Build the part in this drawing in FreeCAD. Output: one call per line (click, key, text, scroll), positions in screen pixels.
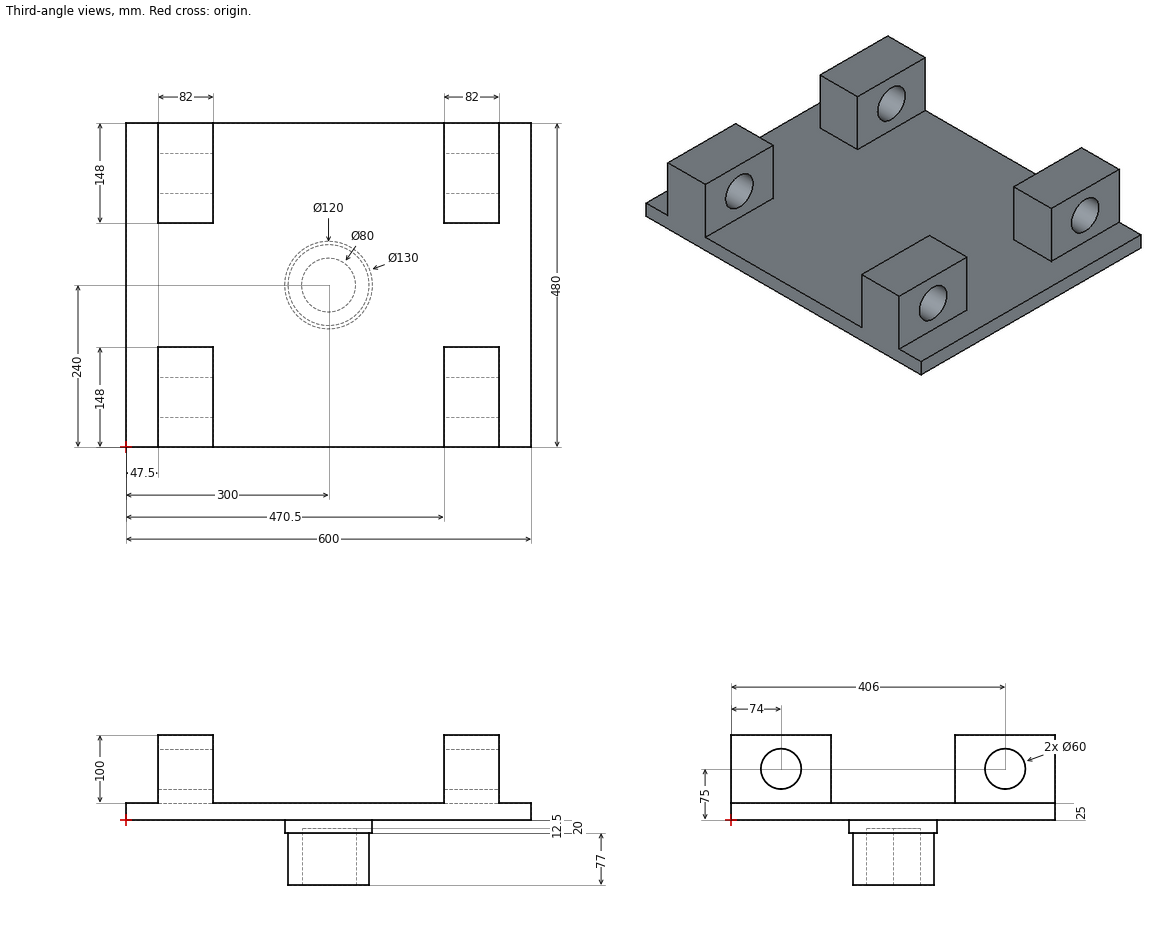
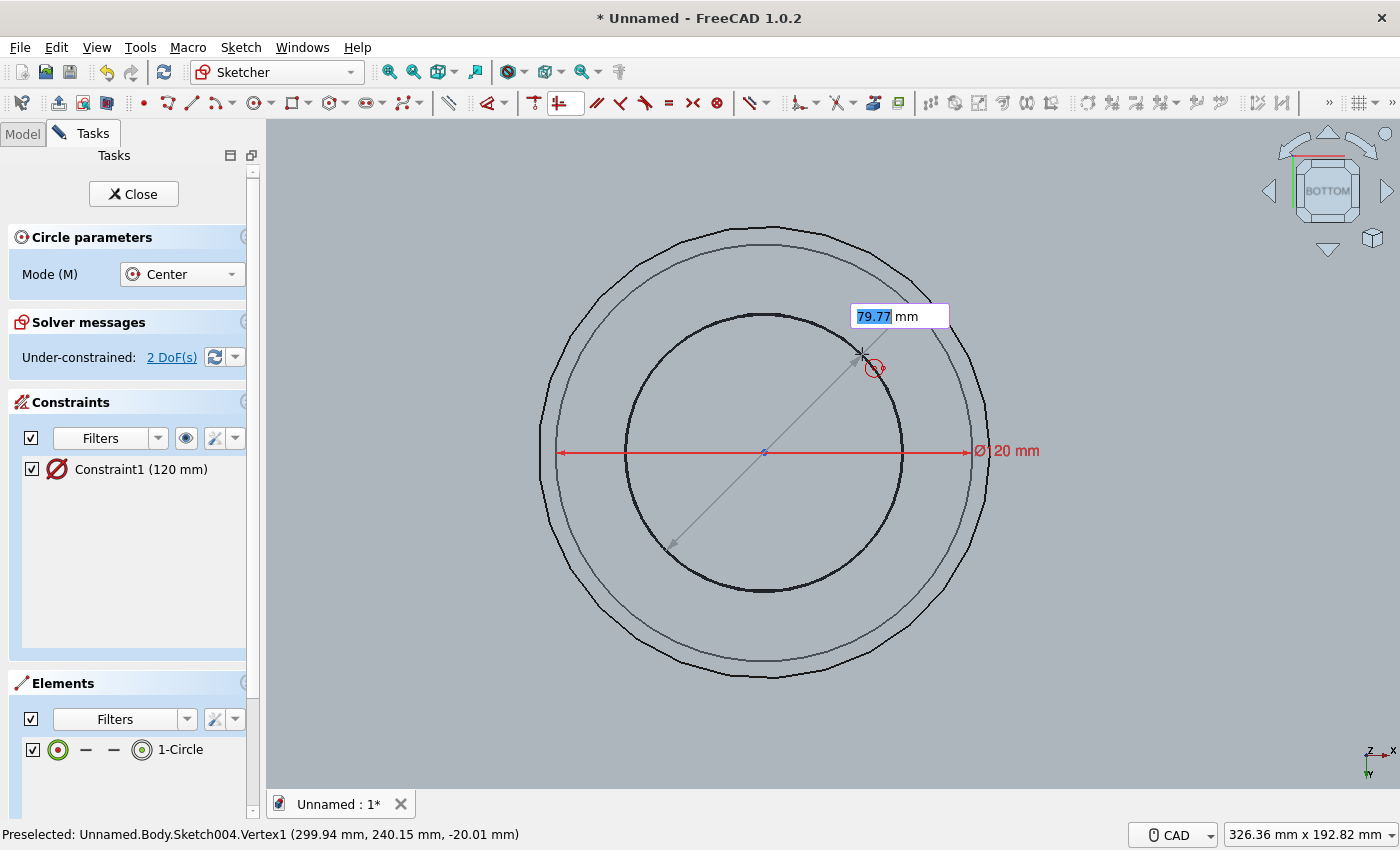
text(80)
key(Return)
key(Escape)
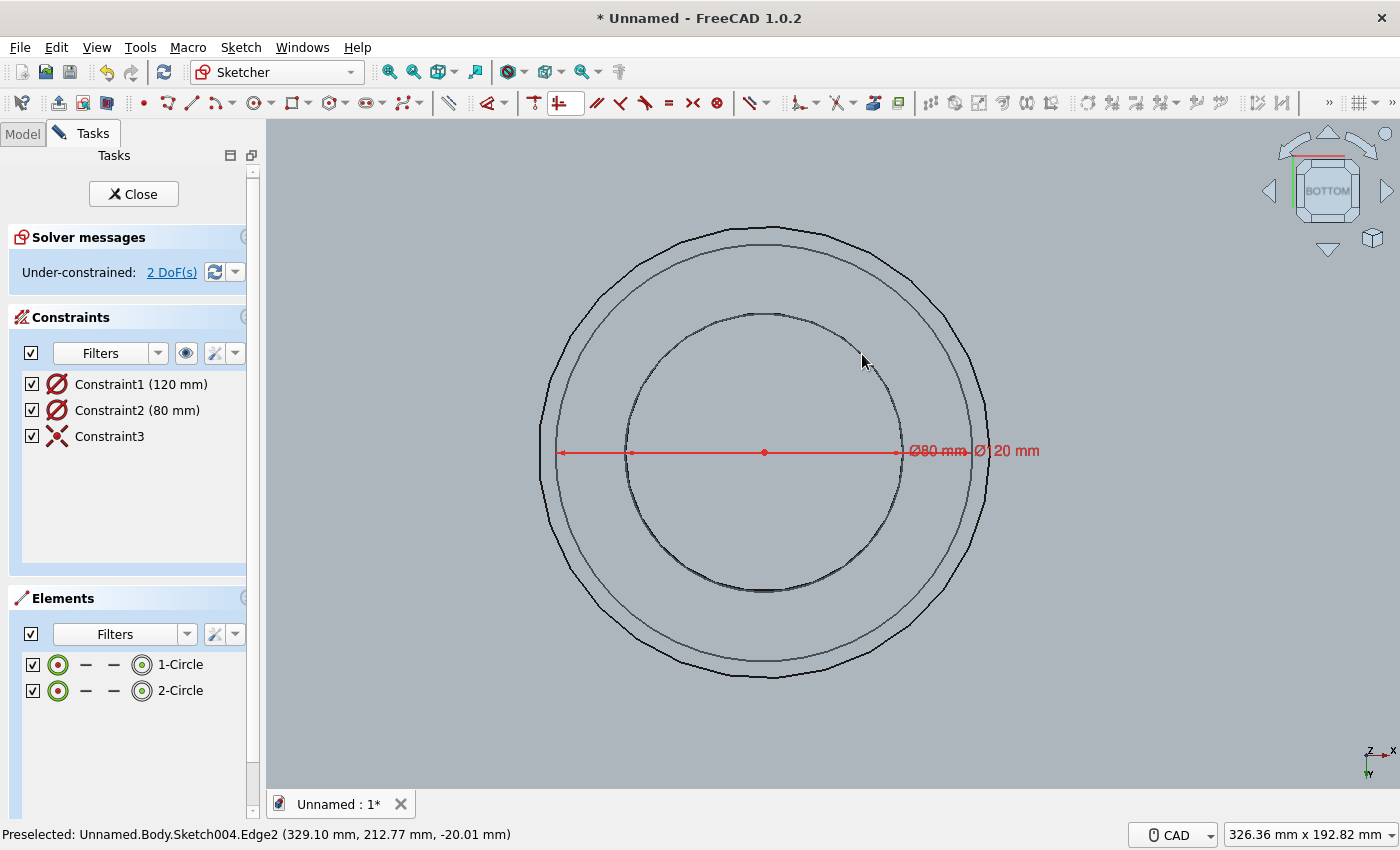
key(d)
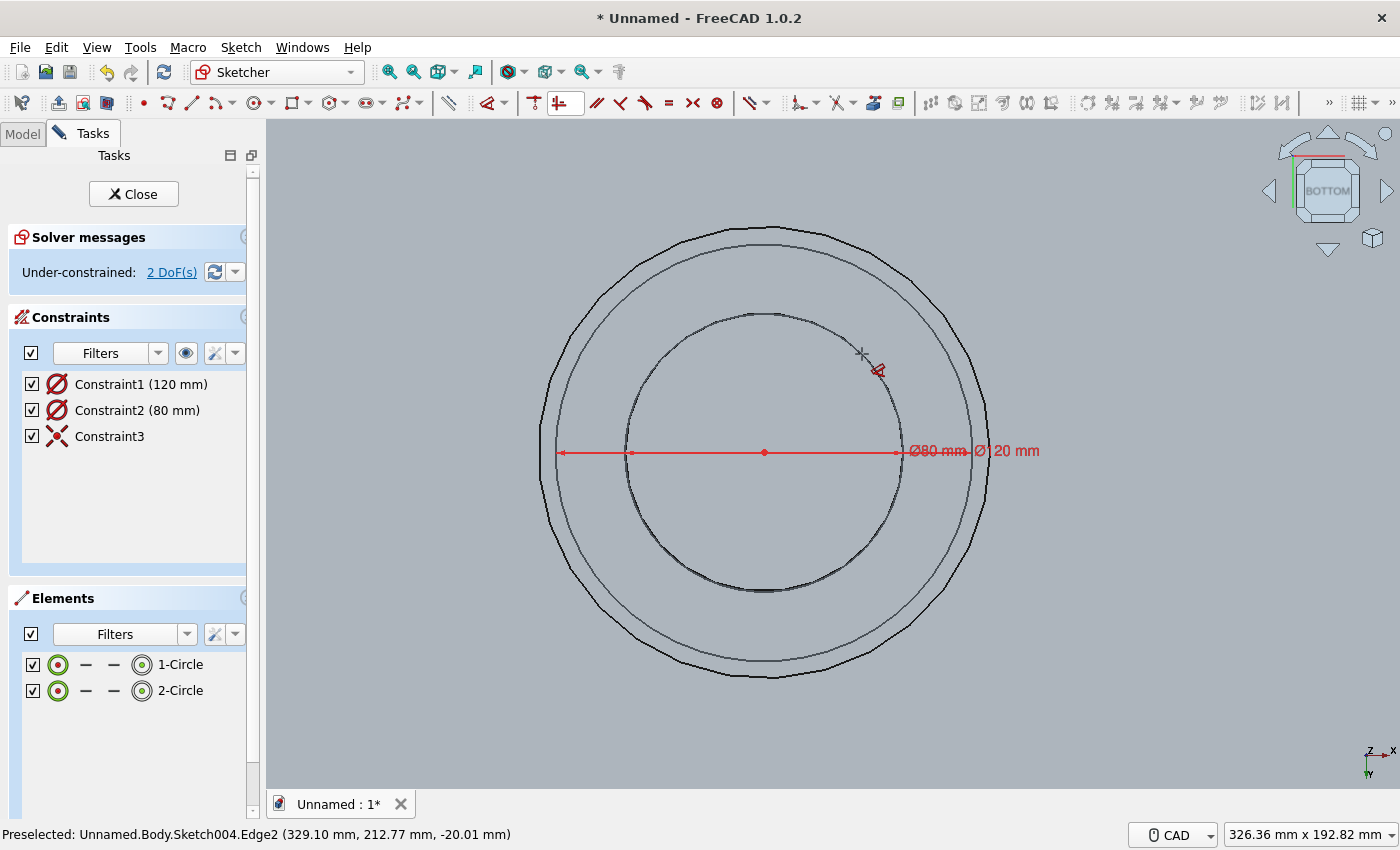
click(764, 453)
click(529, 487)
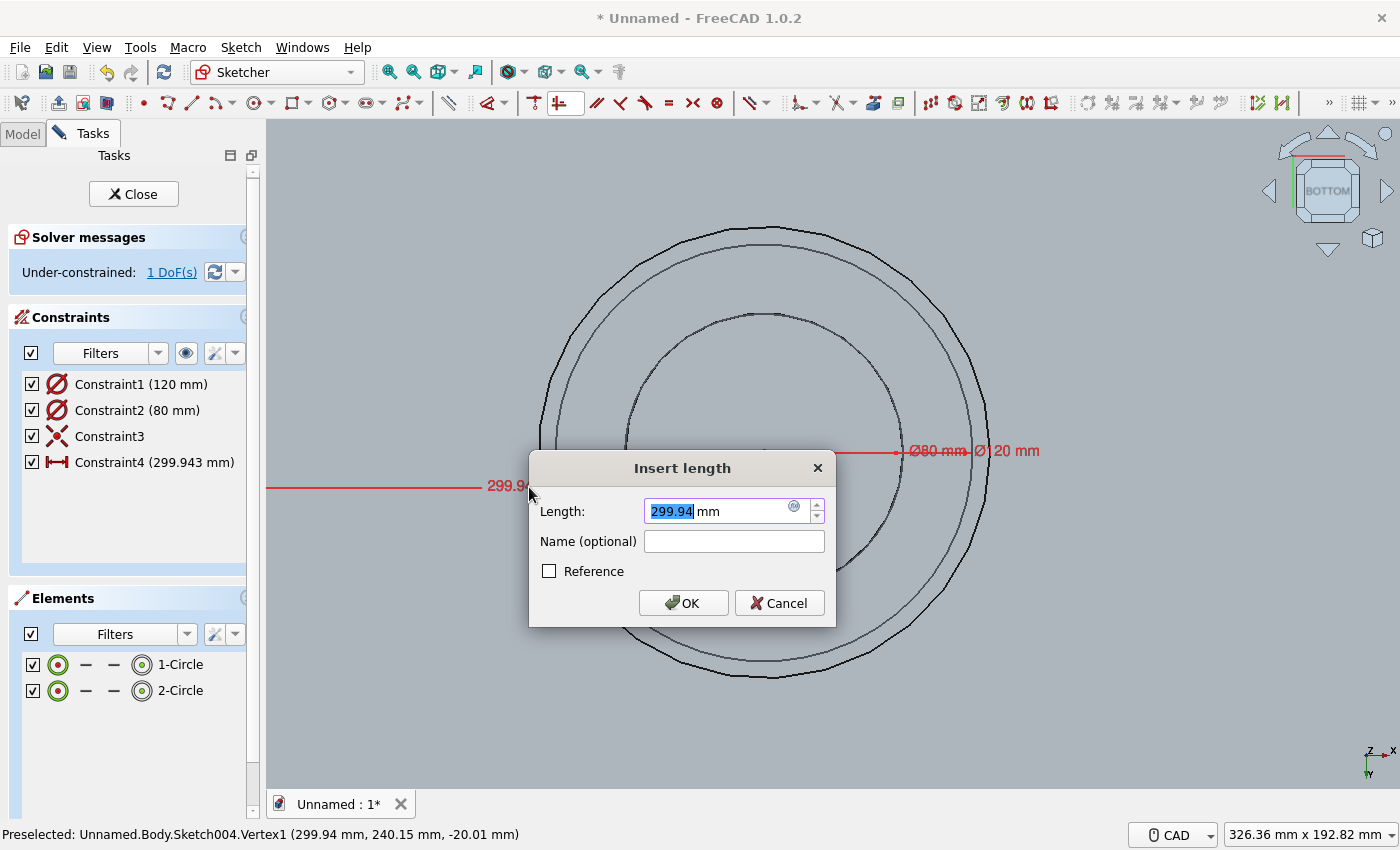
text(300)
key(Return)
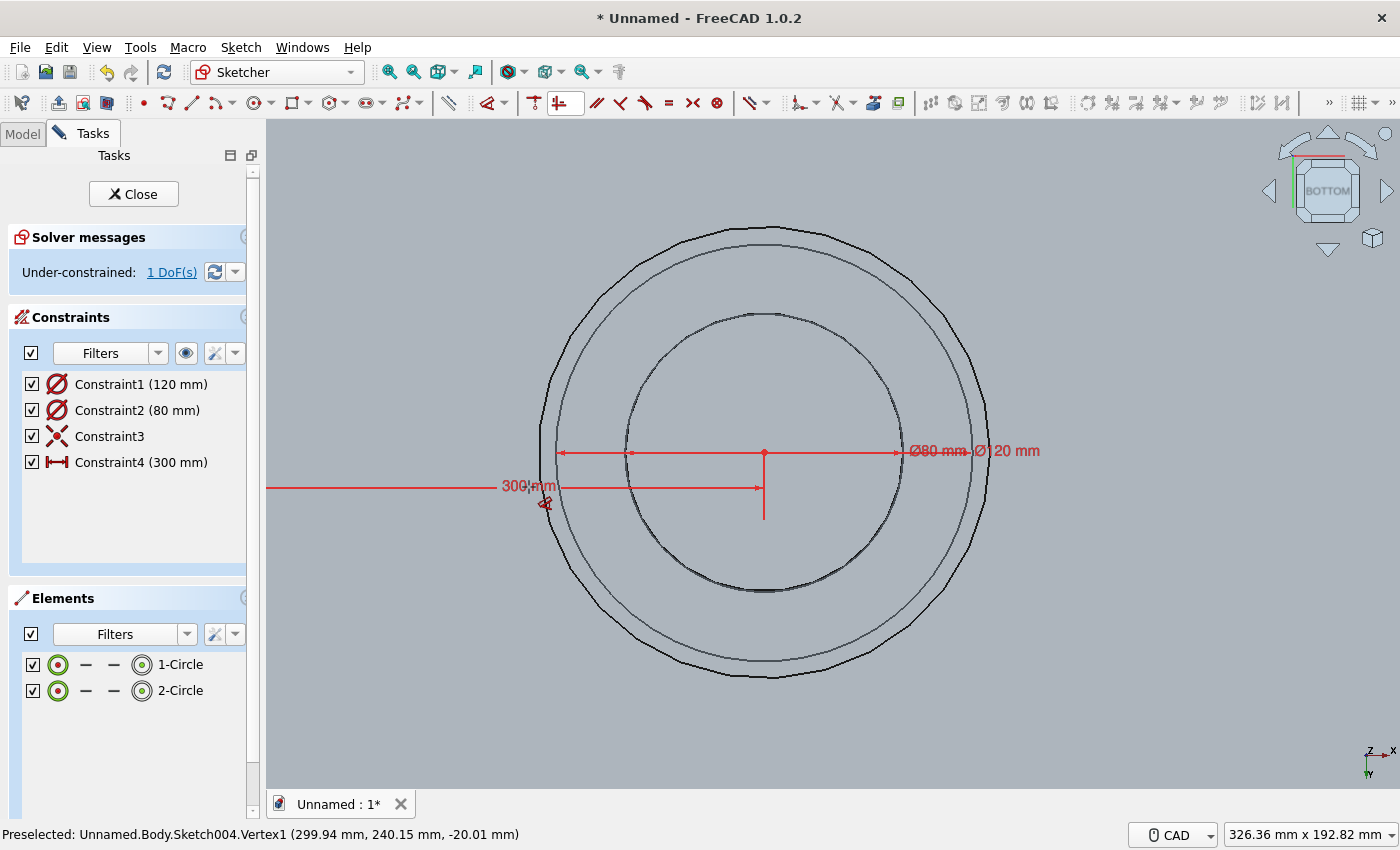
click(764, 453)
click(798, 300)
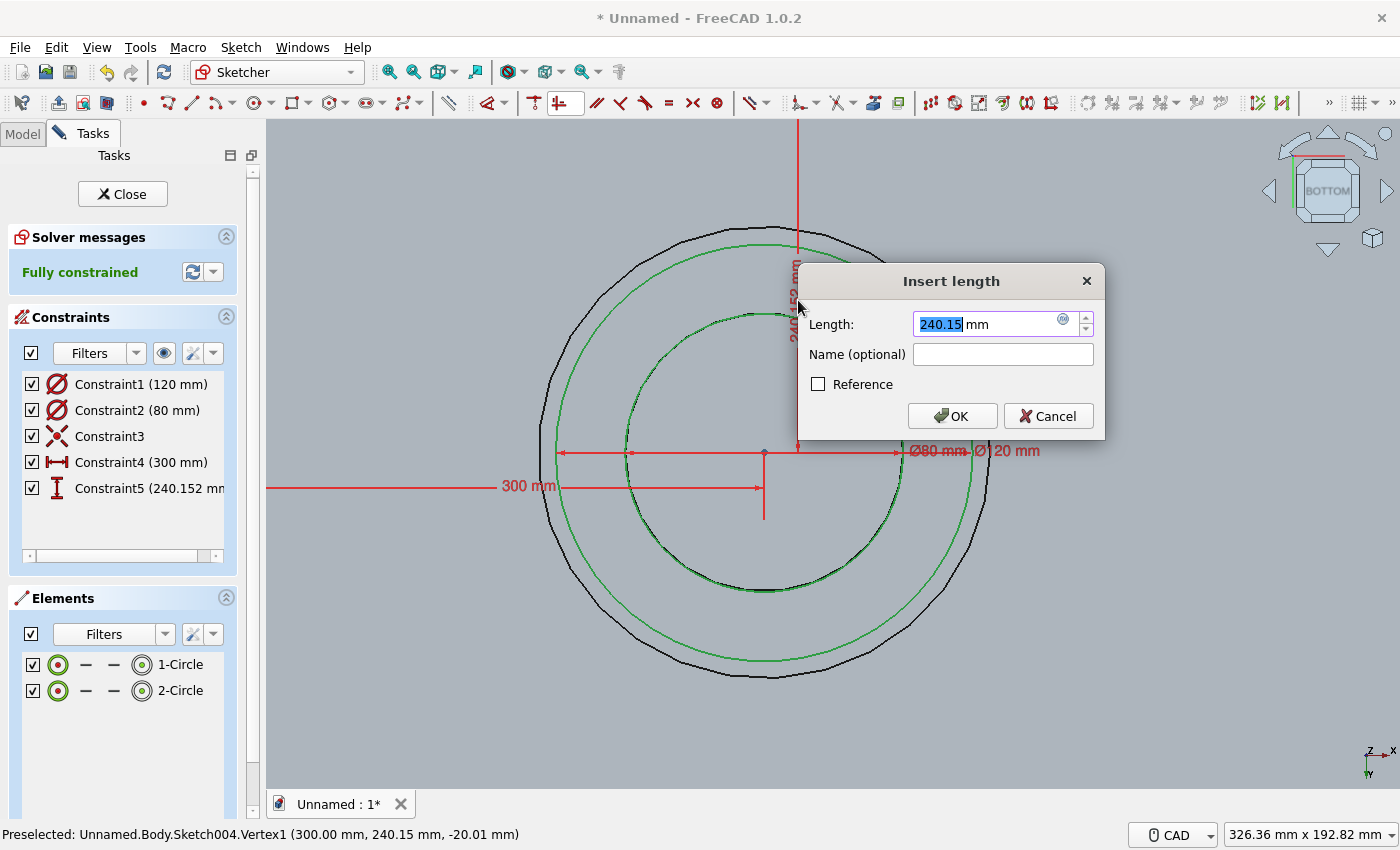
text(240)
key(Return)
key(Escape)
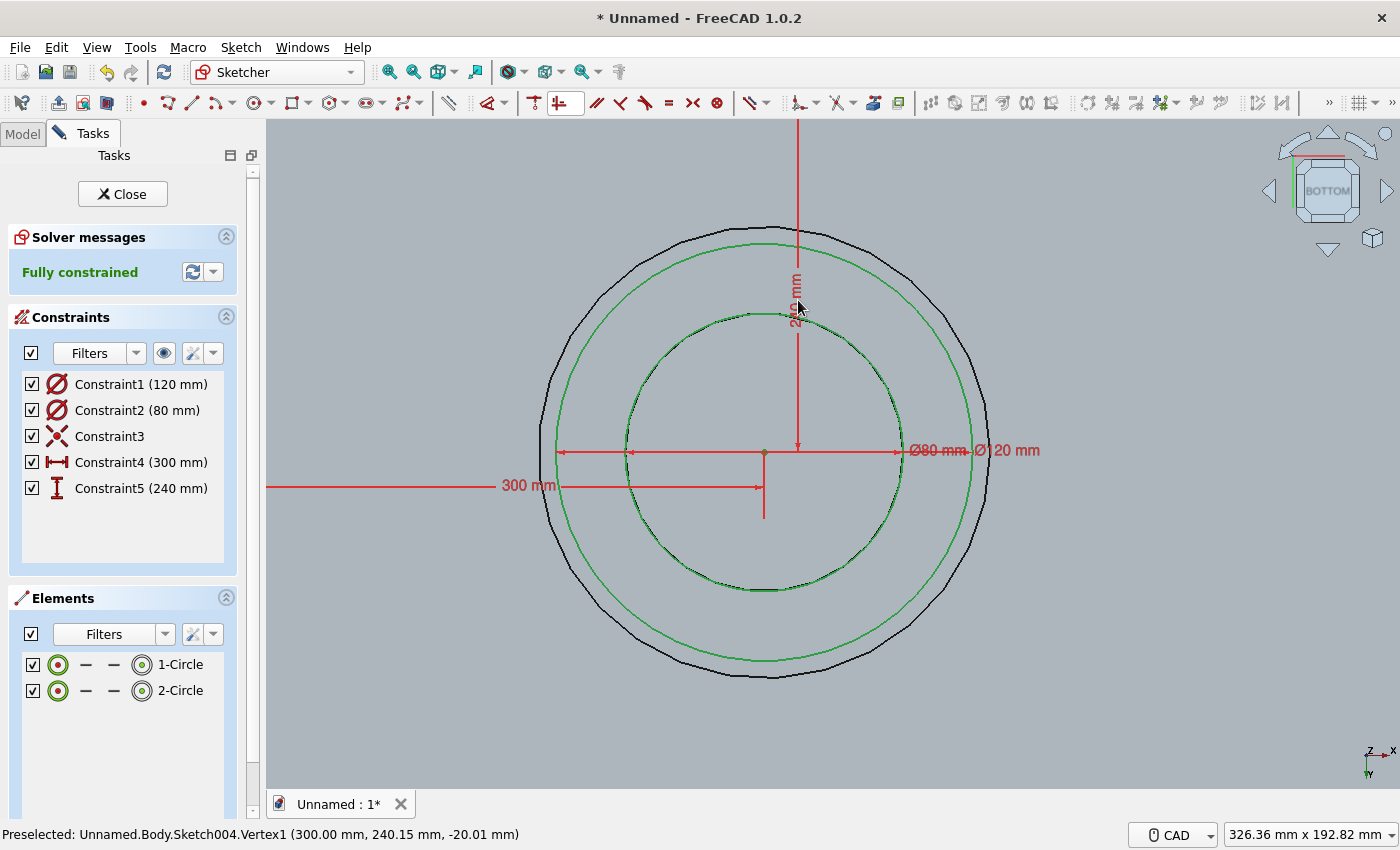
click(123, 194)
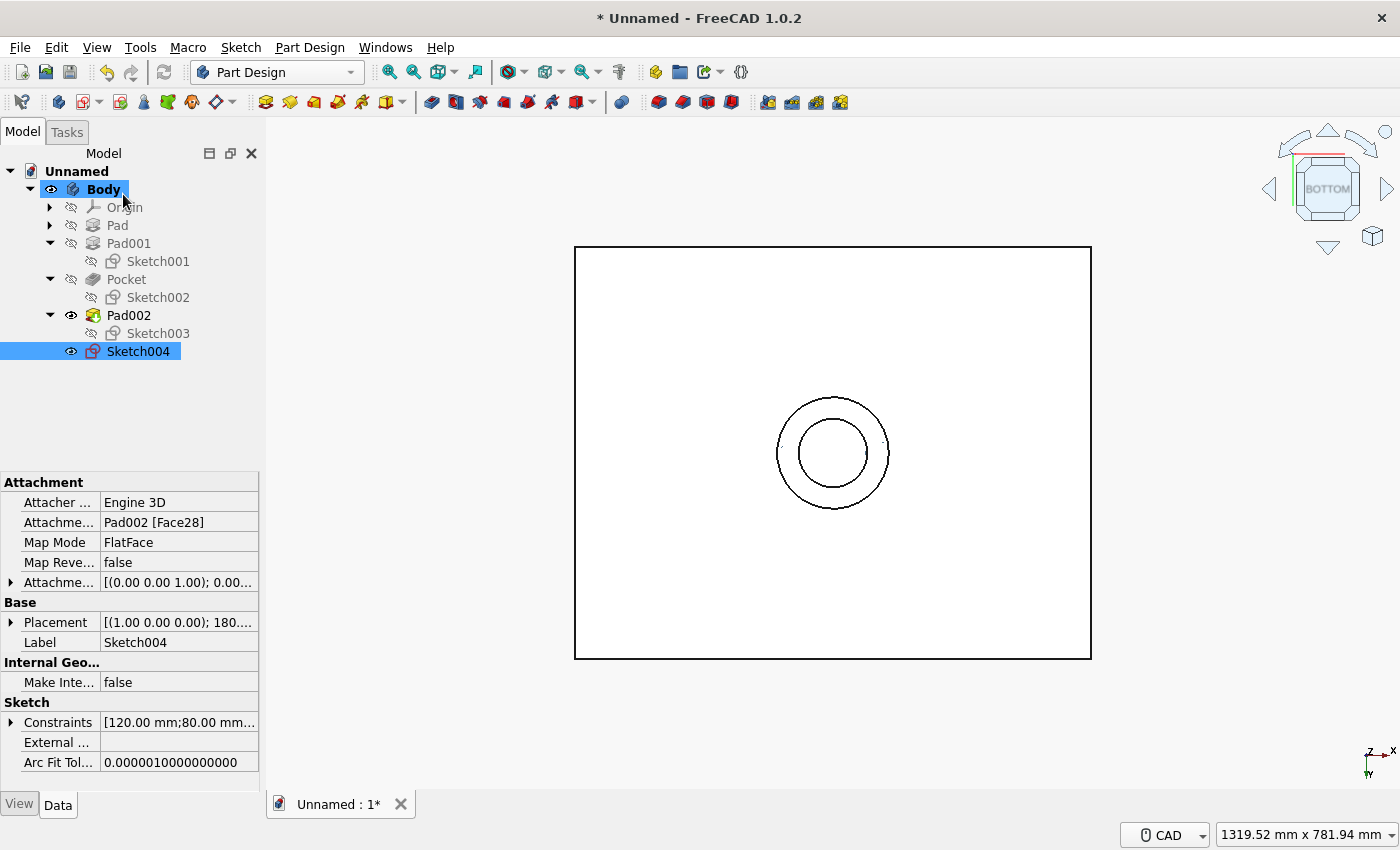
click(266, 102)